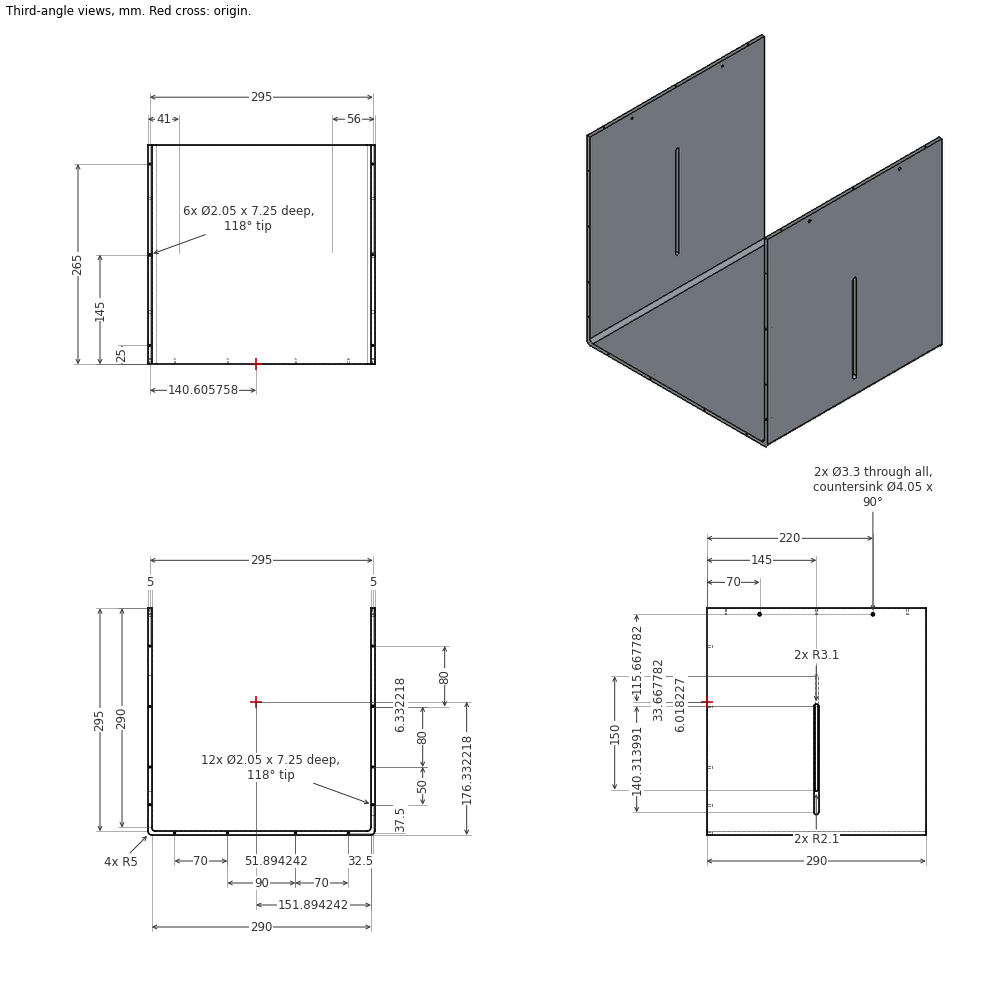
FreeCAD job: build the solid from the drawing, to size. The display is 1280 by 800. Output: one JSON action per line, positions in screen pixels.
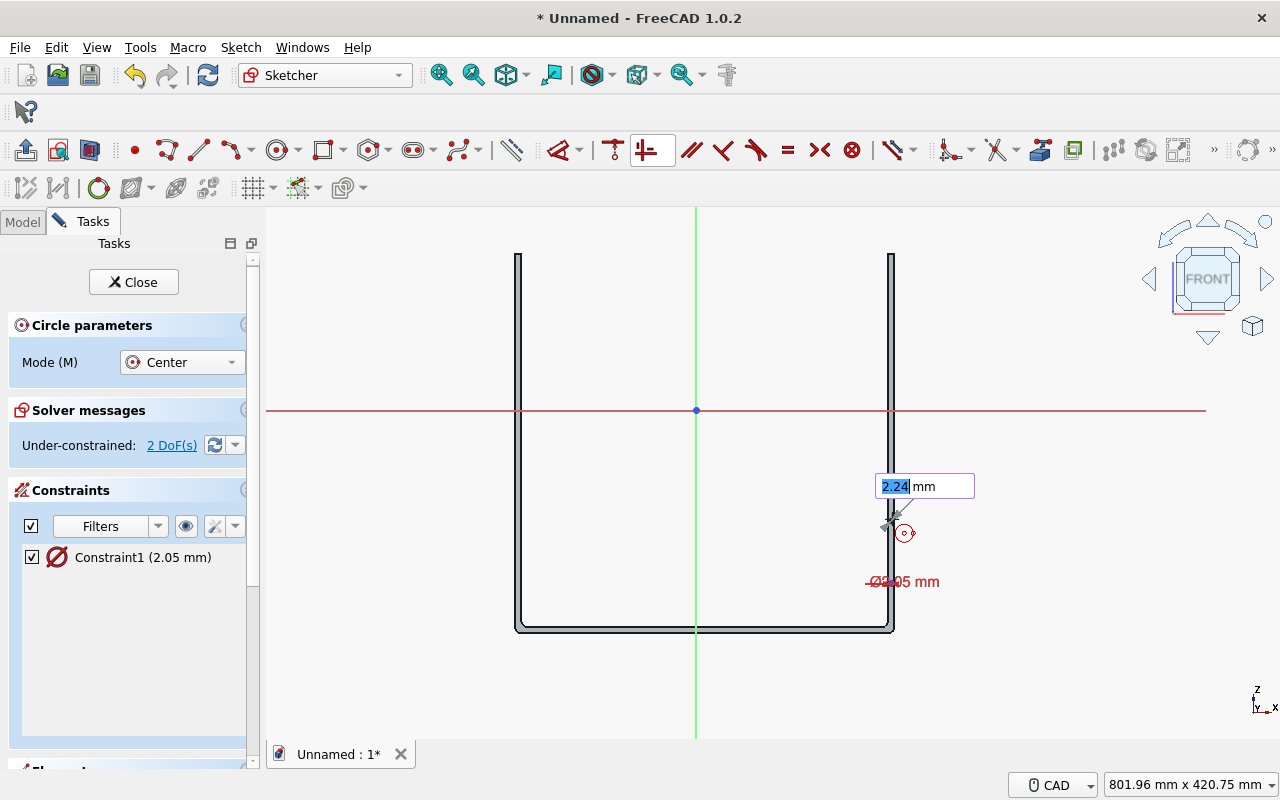
{"action": "type", "text": "2.05"}
{"action": "key", "text": "Return"}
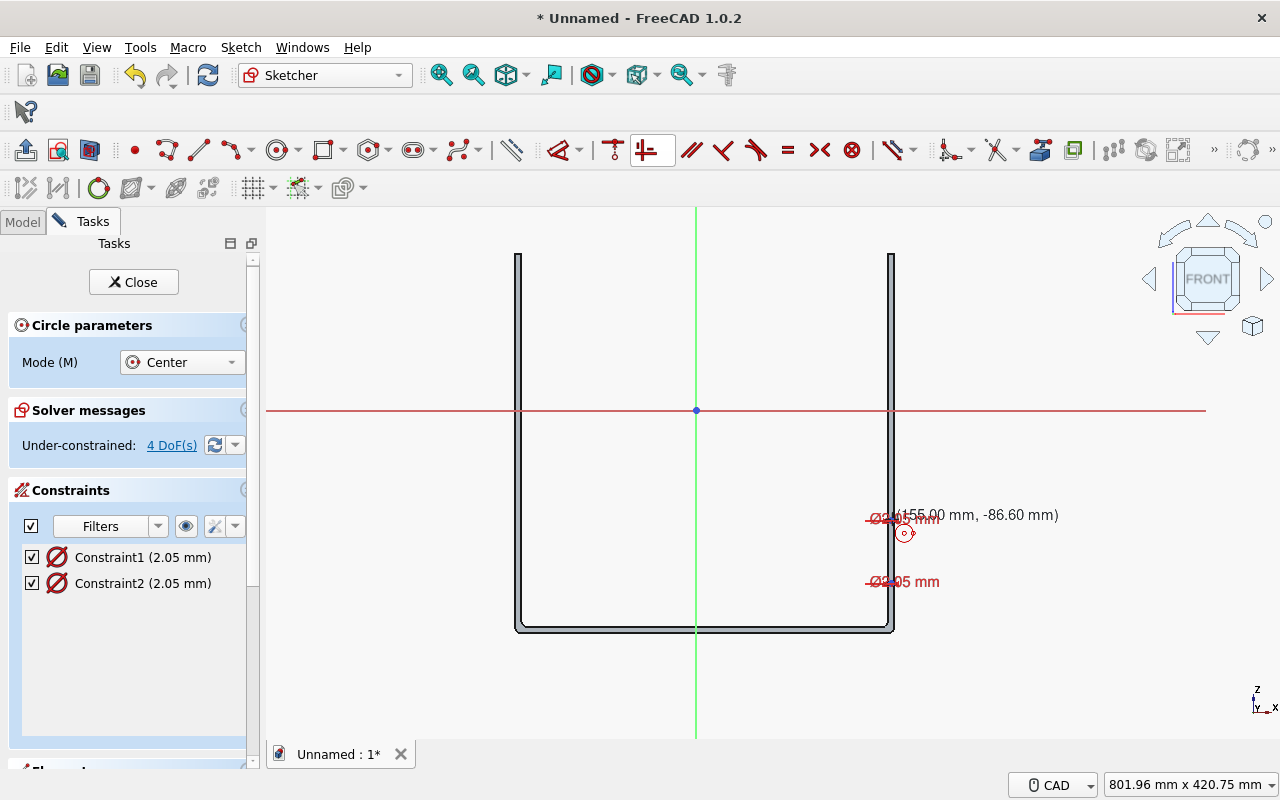
{"action": "scroll", "coordinate": [891, 419], "scroll_direction": "up", "scroll_amount": 15}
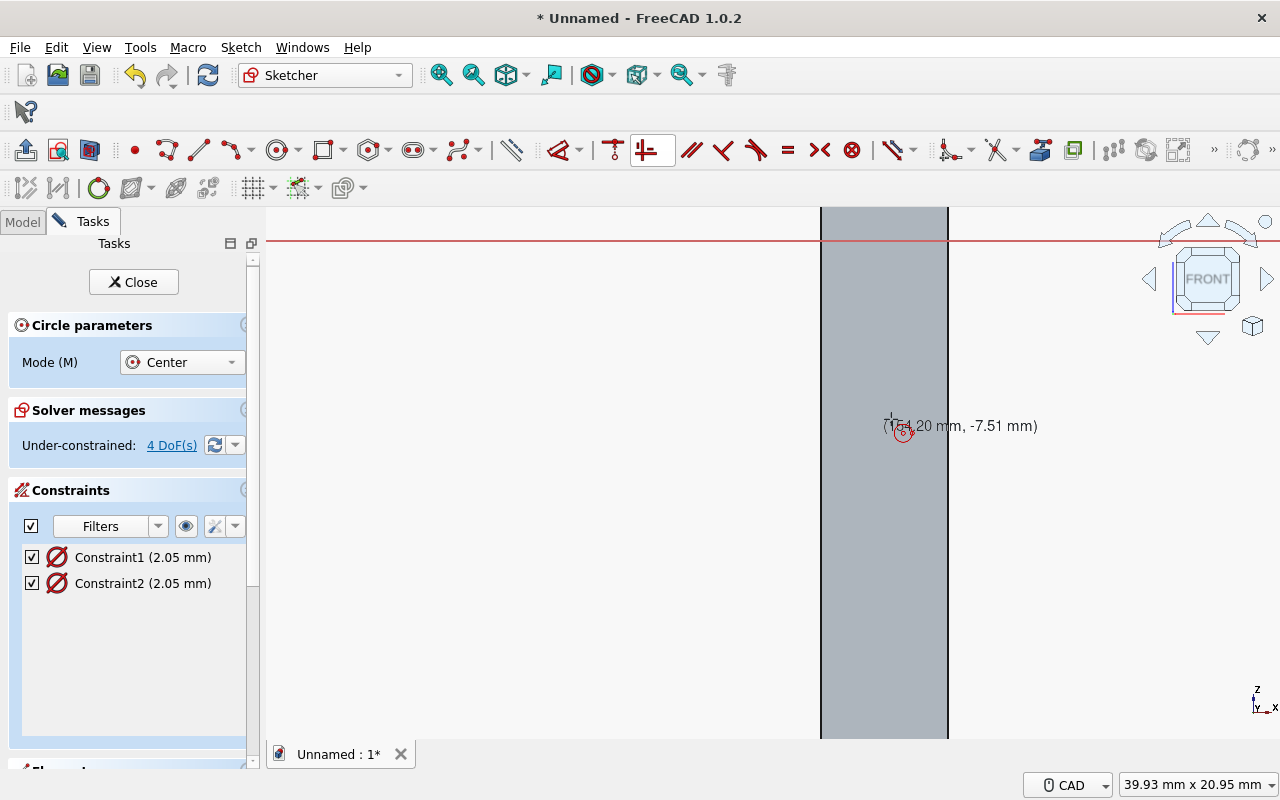
{"action": "scroll", "coordinate": [891, 419], "scroll_direction": "down", "scroll_amount": 15}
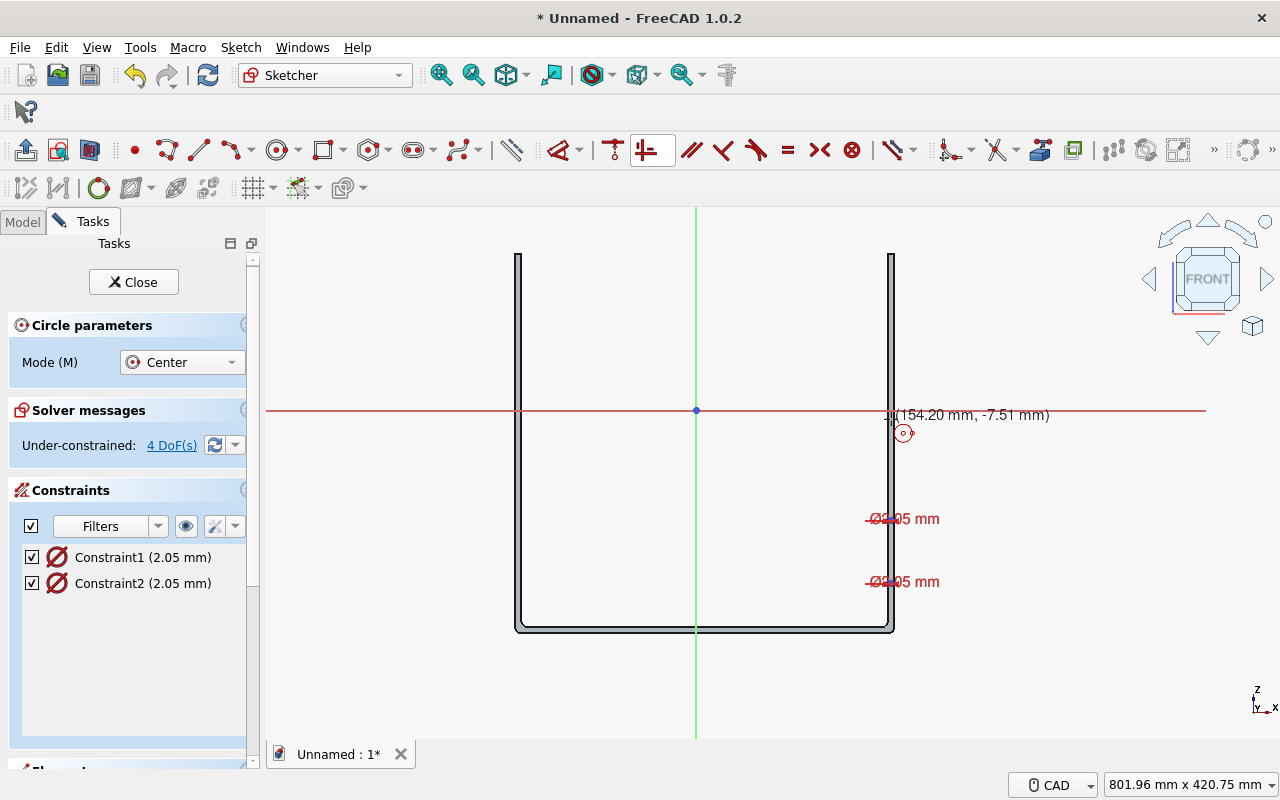
{"action": "scroll", "coordinate": [891, 419], "scroll_direction": "up", "scroll_amount": 4}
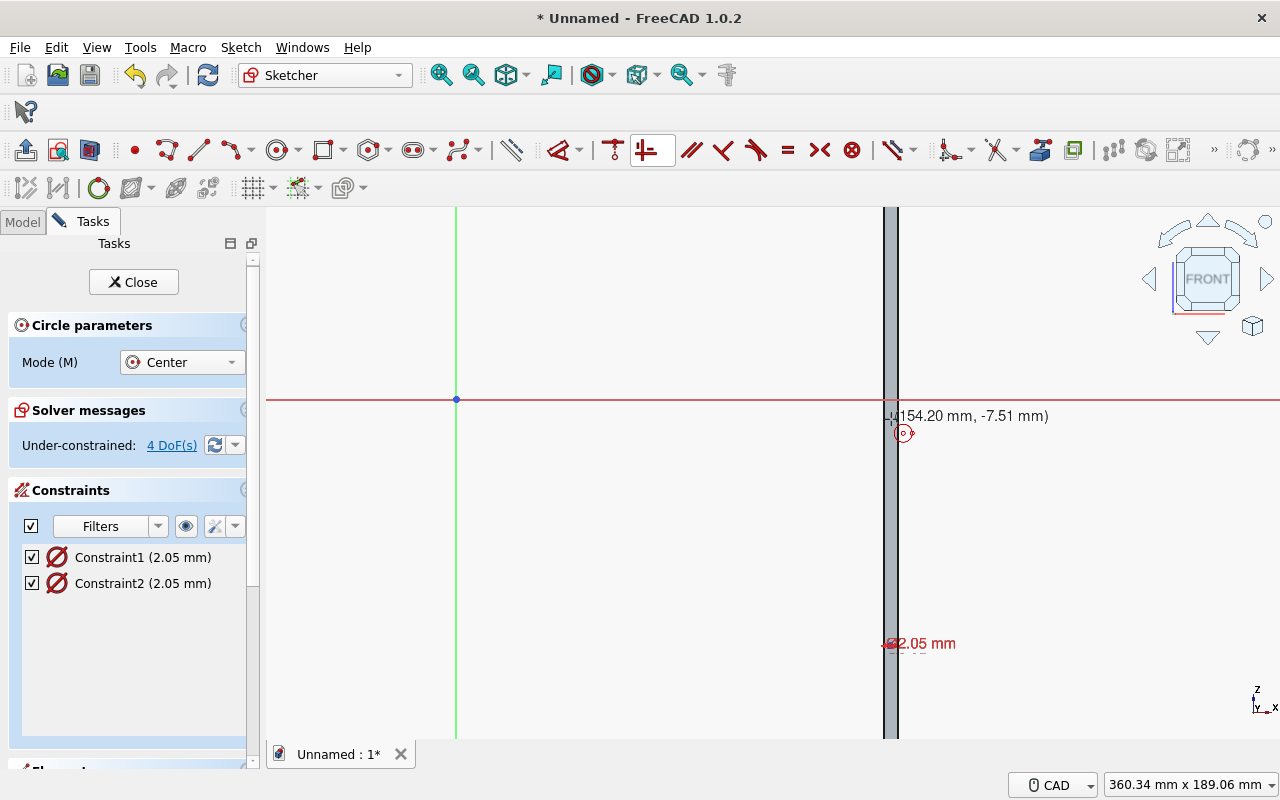
{"action": "left_click", "coordinate": [891, 417]}
{"action": "mouse_move", "coordinate": [893, 415]}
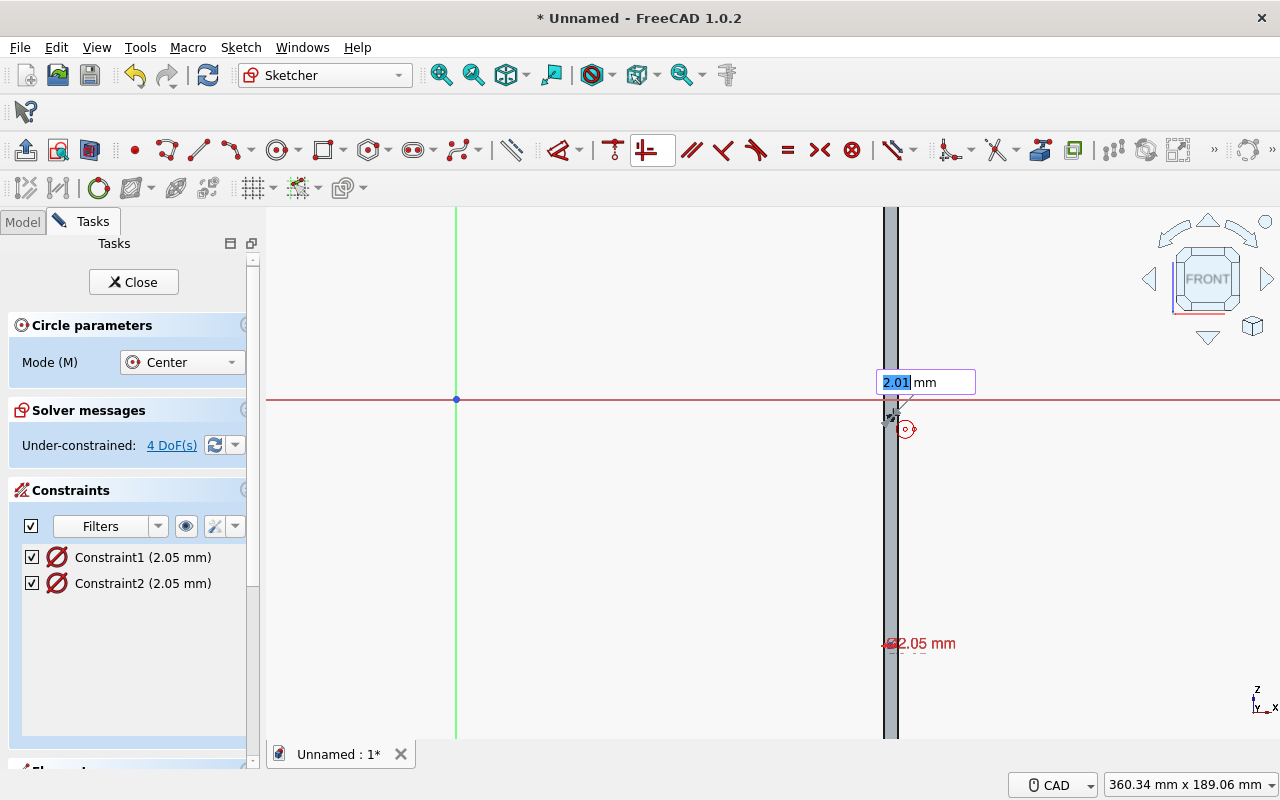
{"action": "type", "text": "2.05"}
{"action": "key", "text": "Return"}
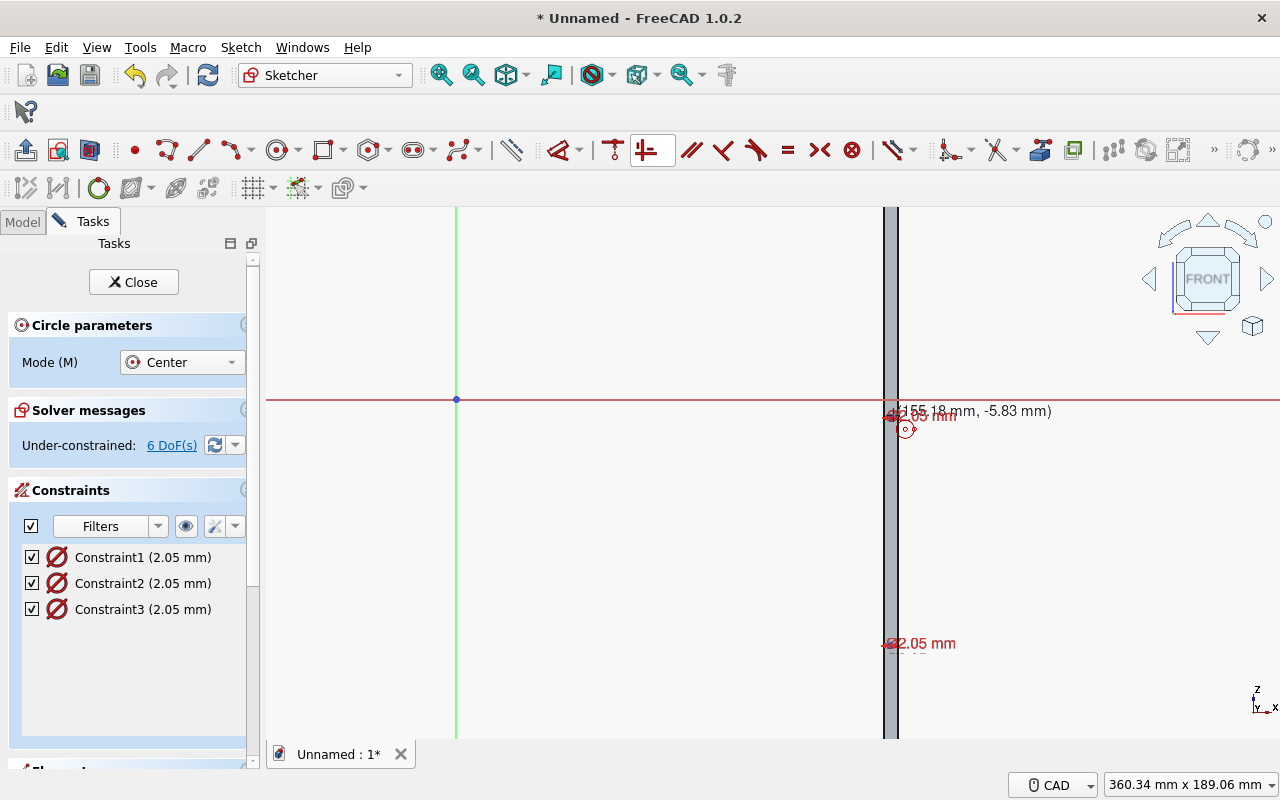
{"action": "scroll", "coordinate": [891, 418], "scroll_direction": "down", "scroll_amount": 4}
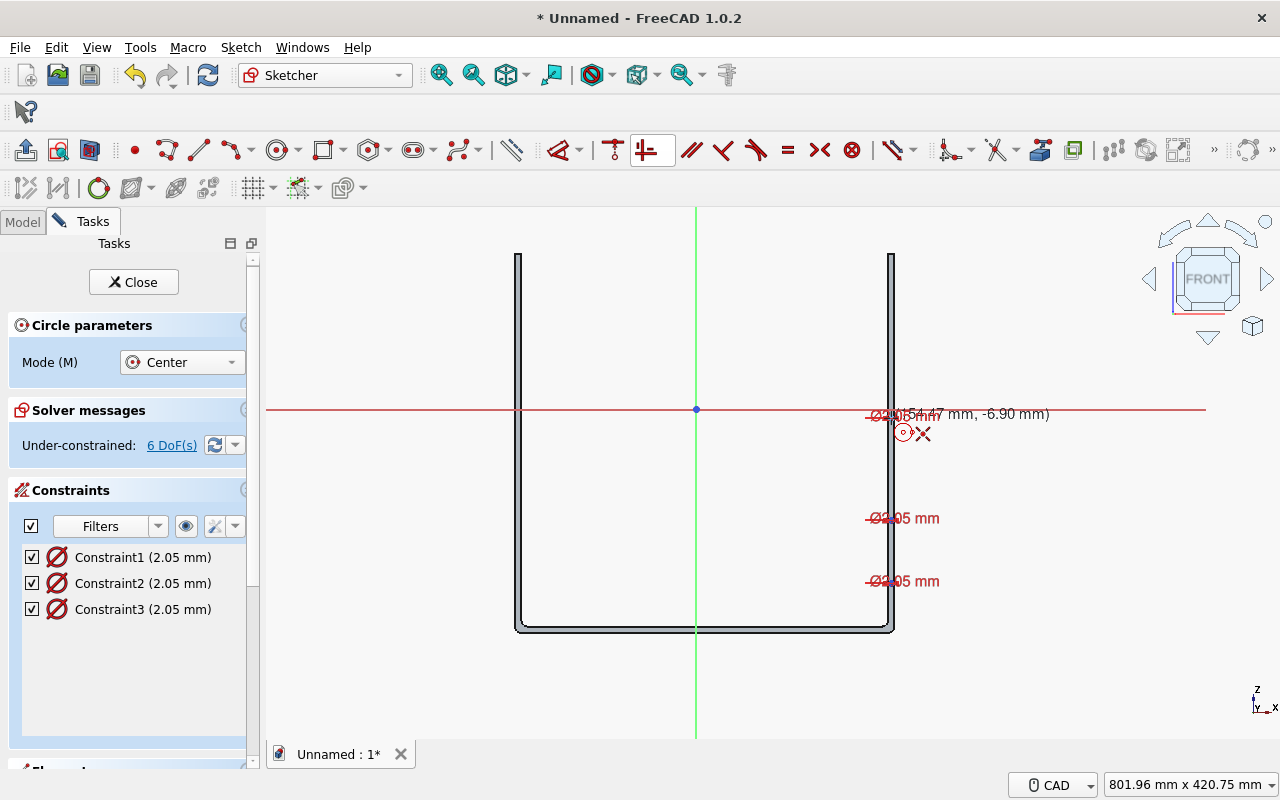
{"action": "scroll", "coordinate": [891, 317], "scroll_direction": "up", "scroll_amount": 15}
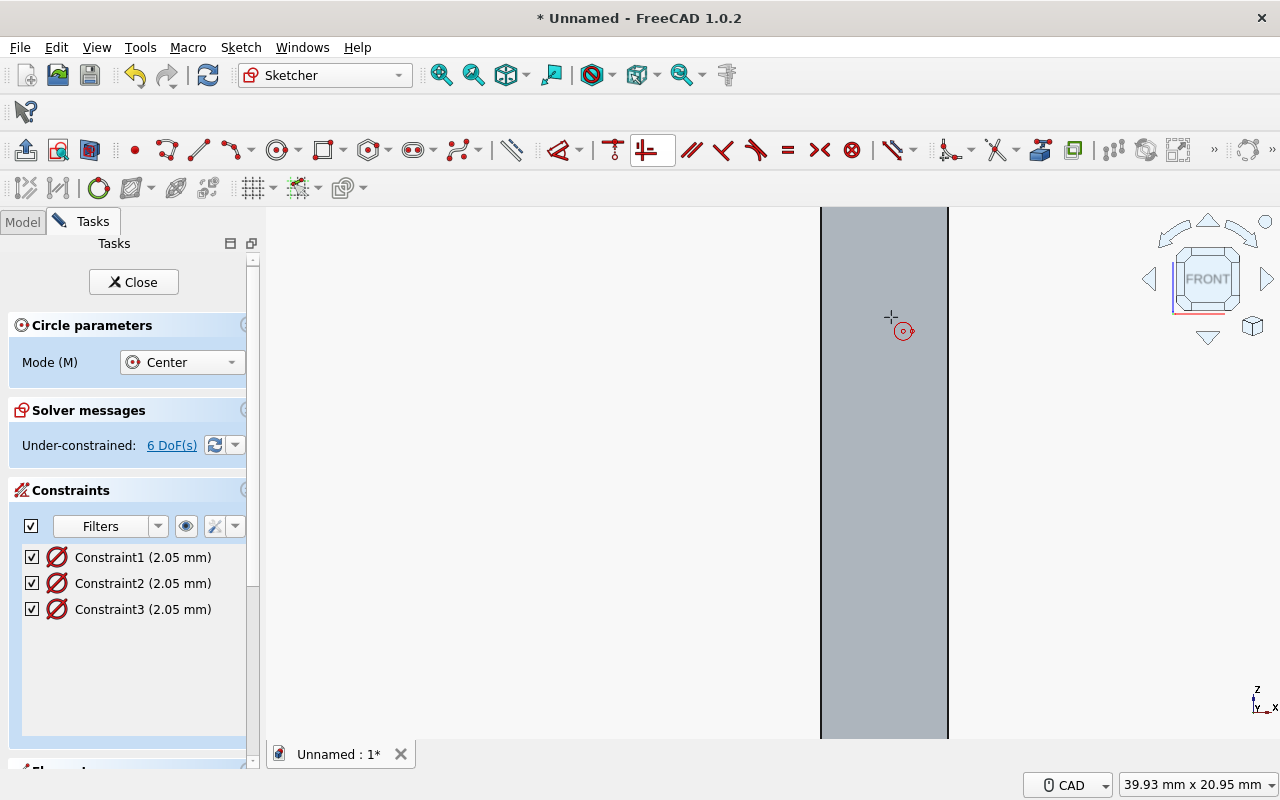
{"action": "scroll", "coordinate": [891, 317], "scroll_direction": "down", "scroll_amount": 15}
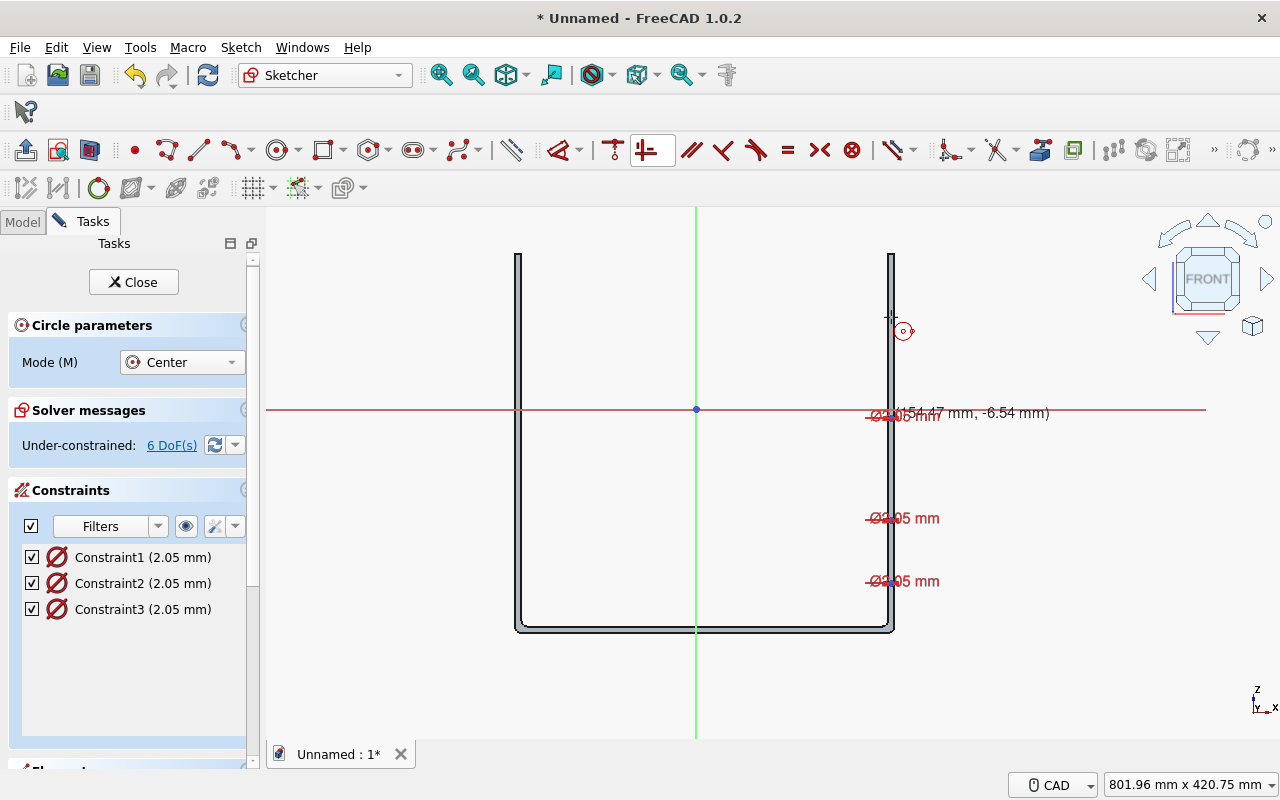
{"action": "left_click", "coordinate": [891, 317]}
{"action": "mouse_move", "coordinate": [892, 316]}